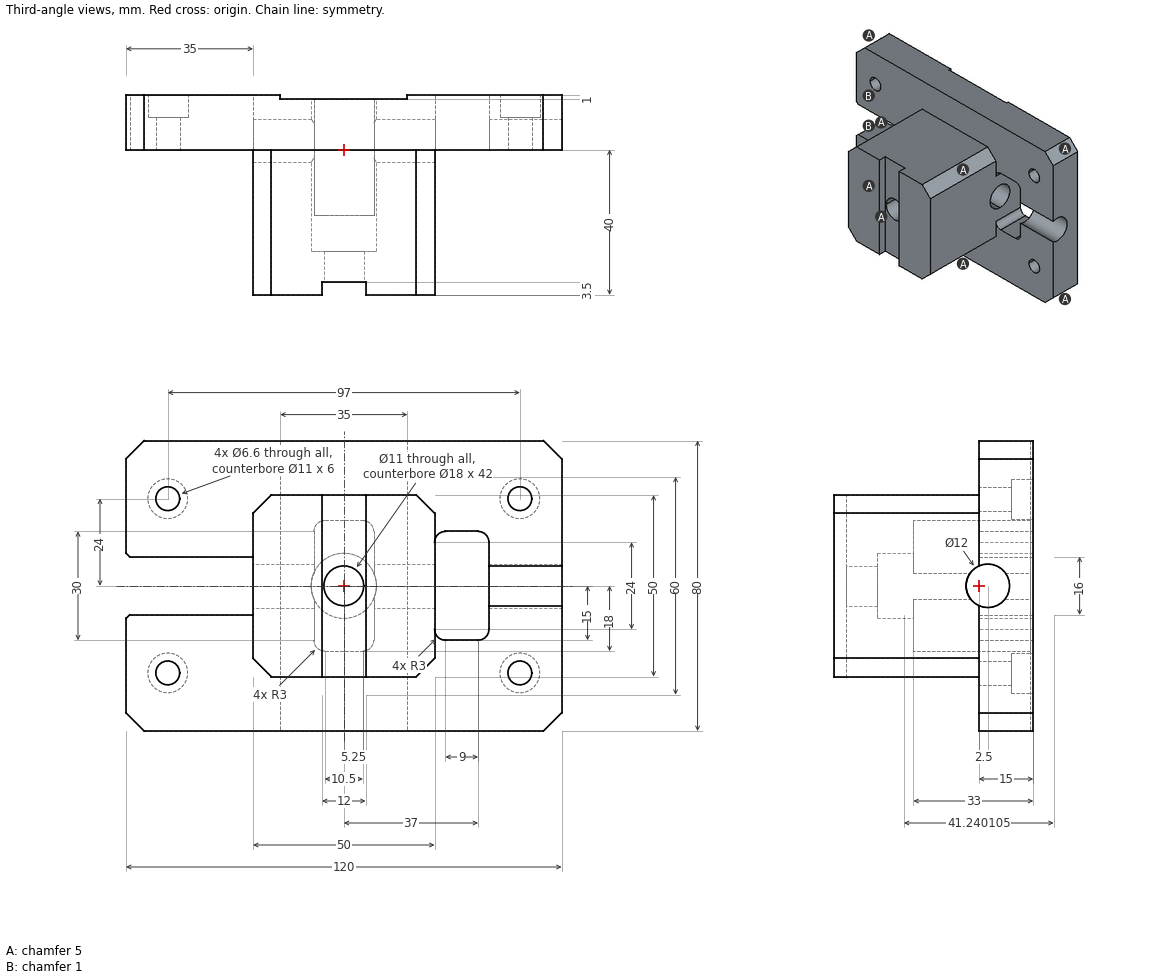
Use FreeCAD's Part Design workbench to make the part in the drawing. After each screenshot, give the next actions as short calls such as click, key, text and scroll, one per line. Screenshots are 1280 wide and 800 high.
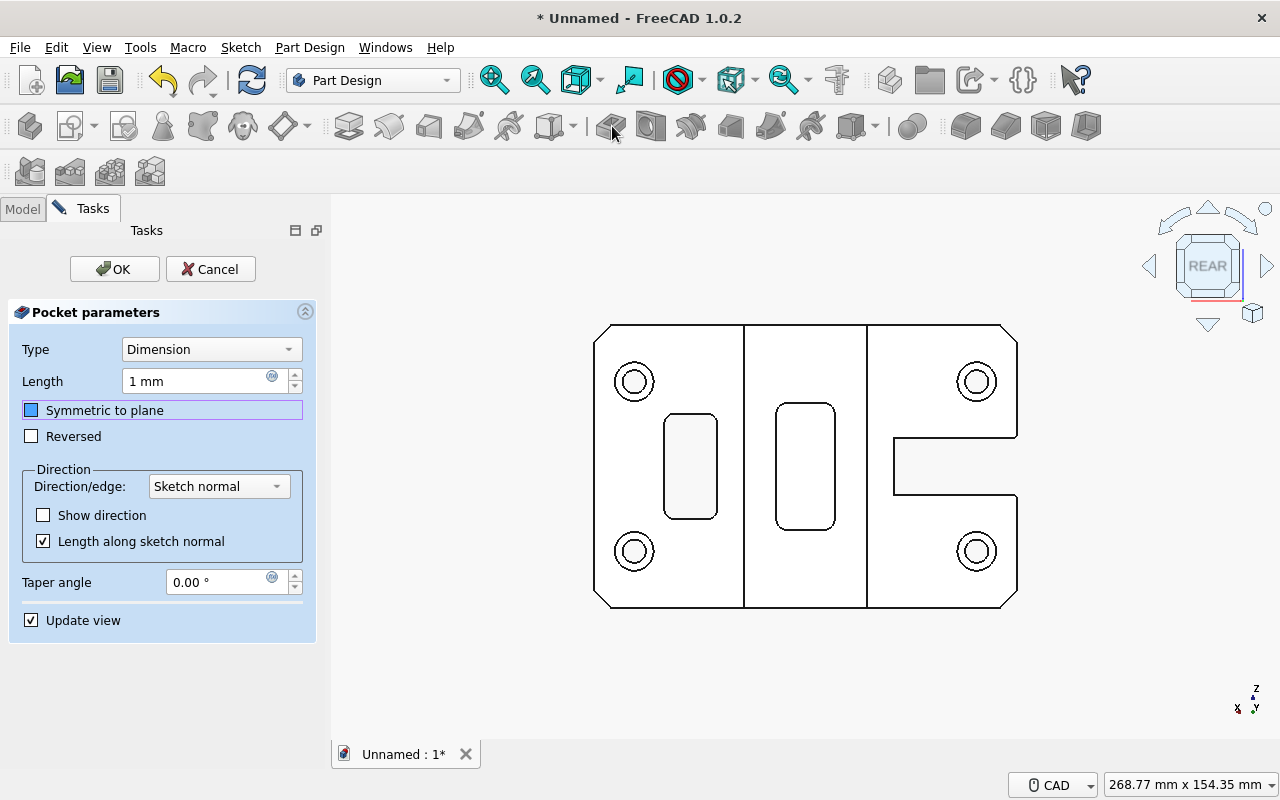
click(115, 269)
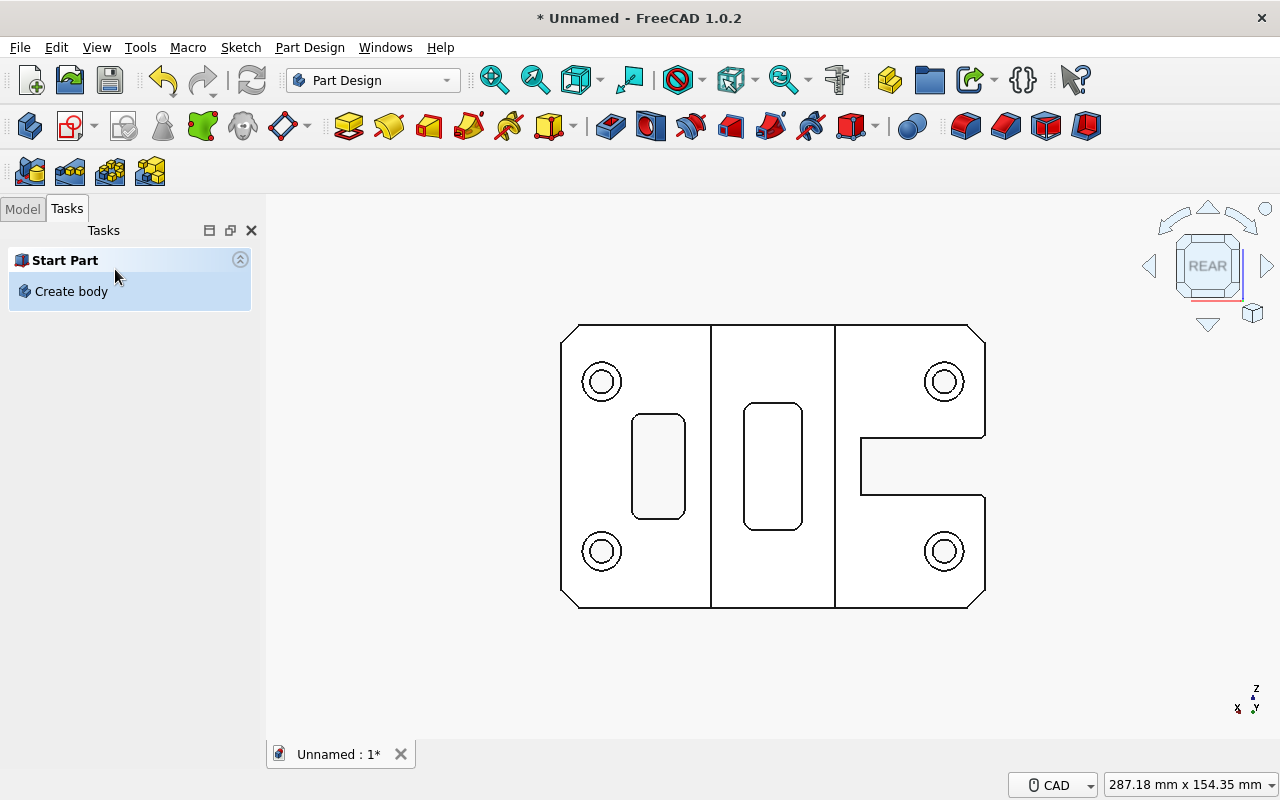
click(738, 546)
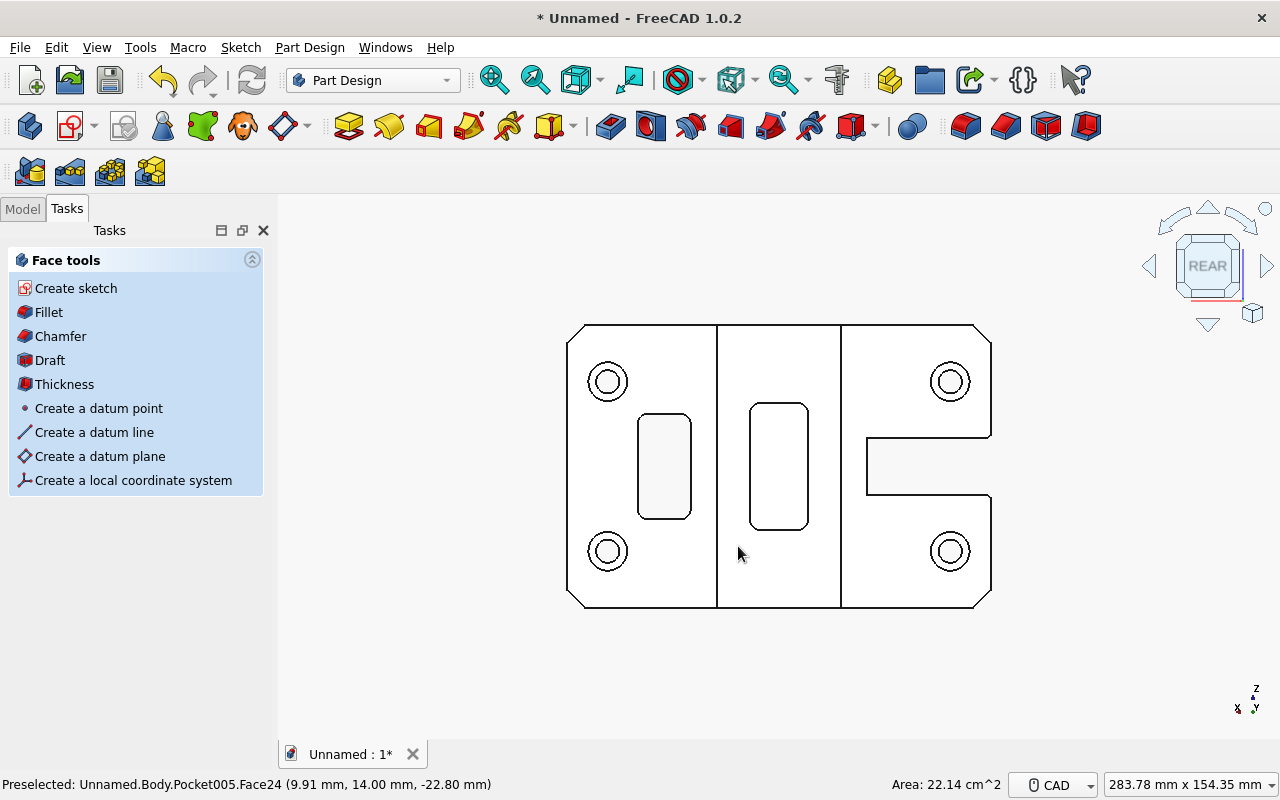
click(70, 126)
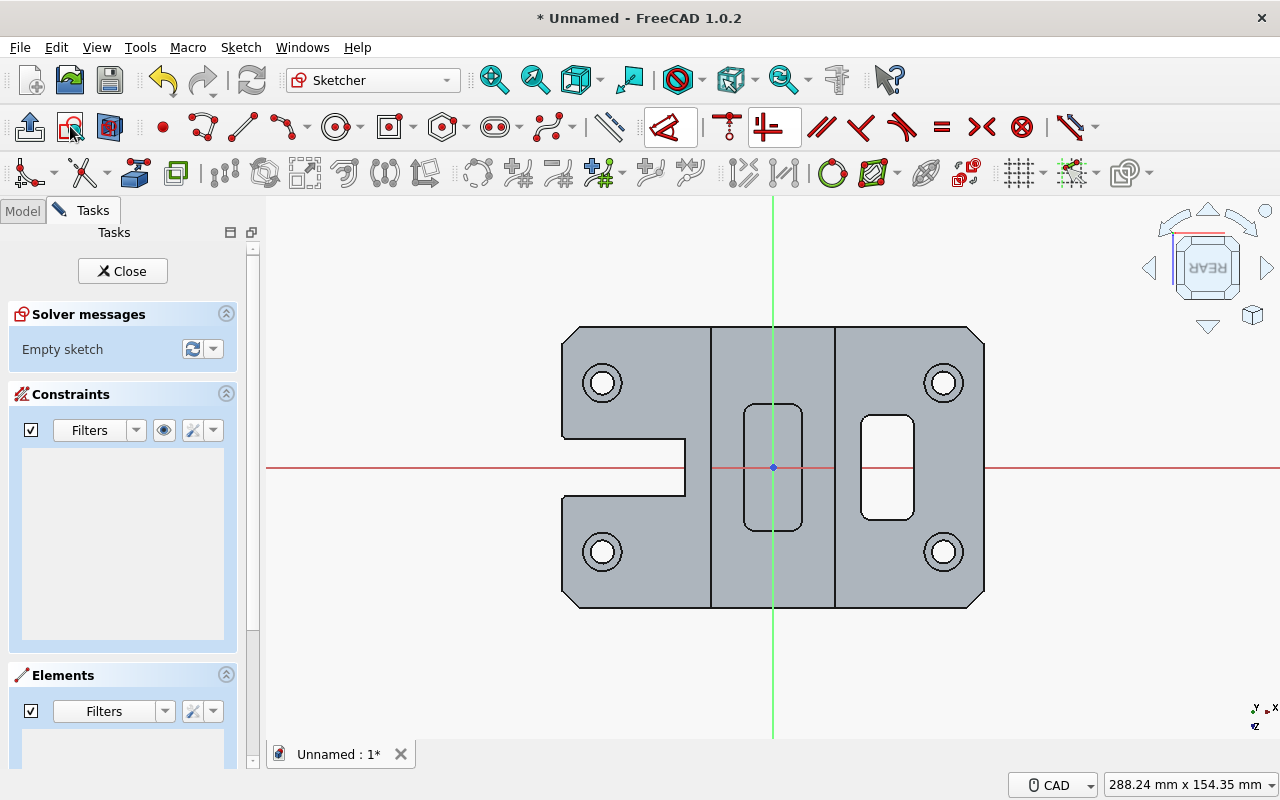
scroll(782, 467, up, 11)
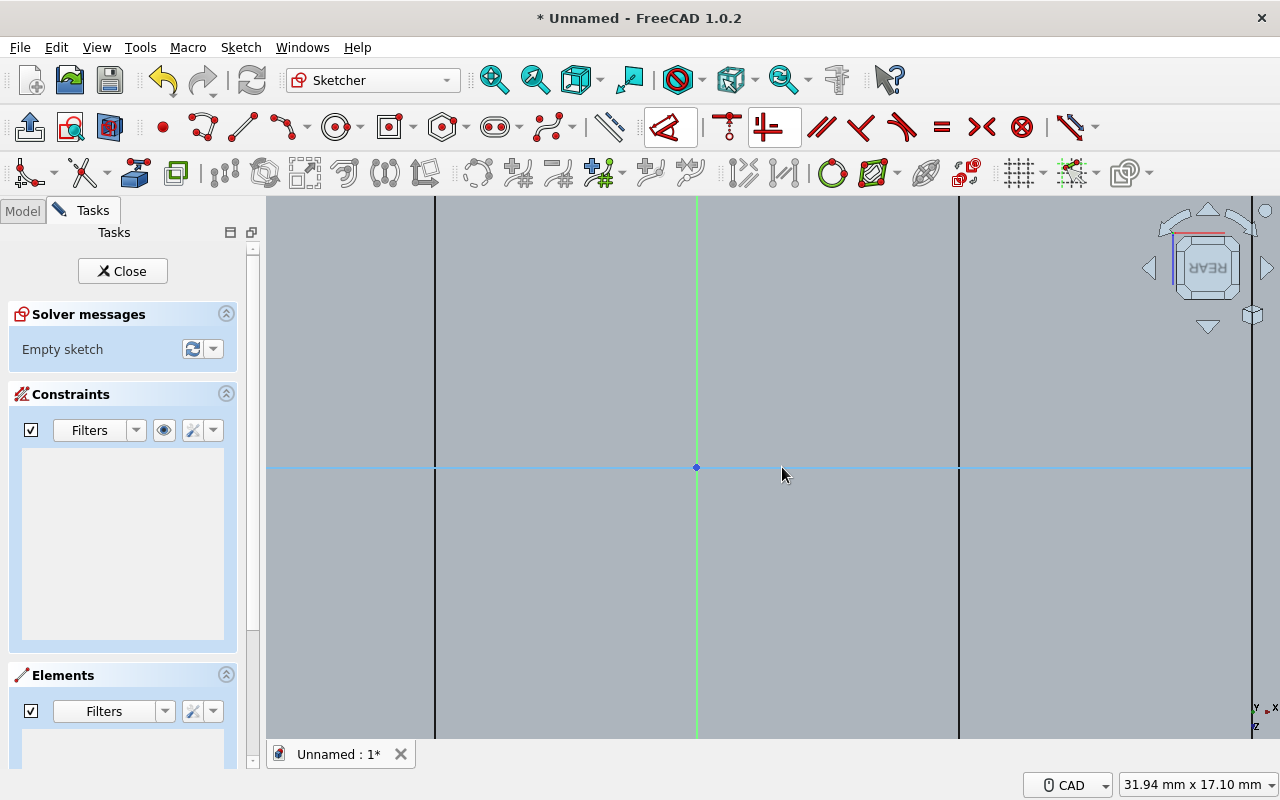
click(336, 128)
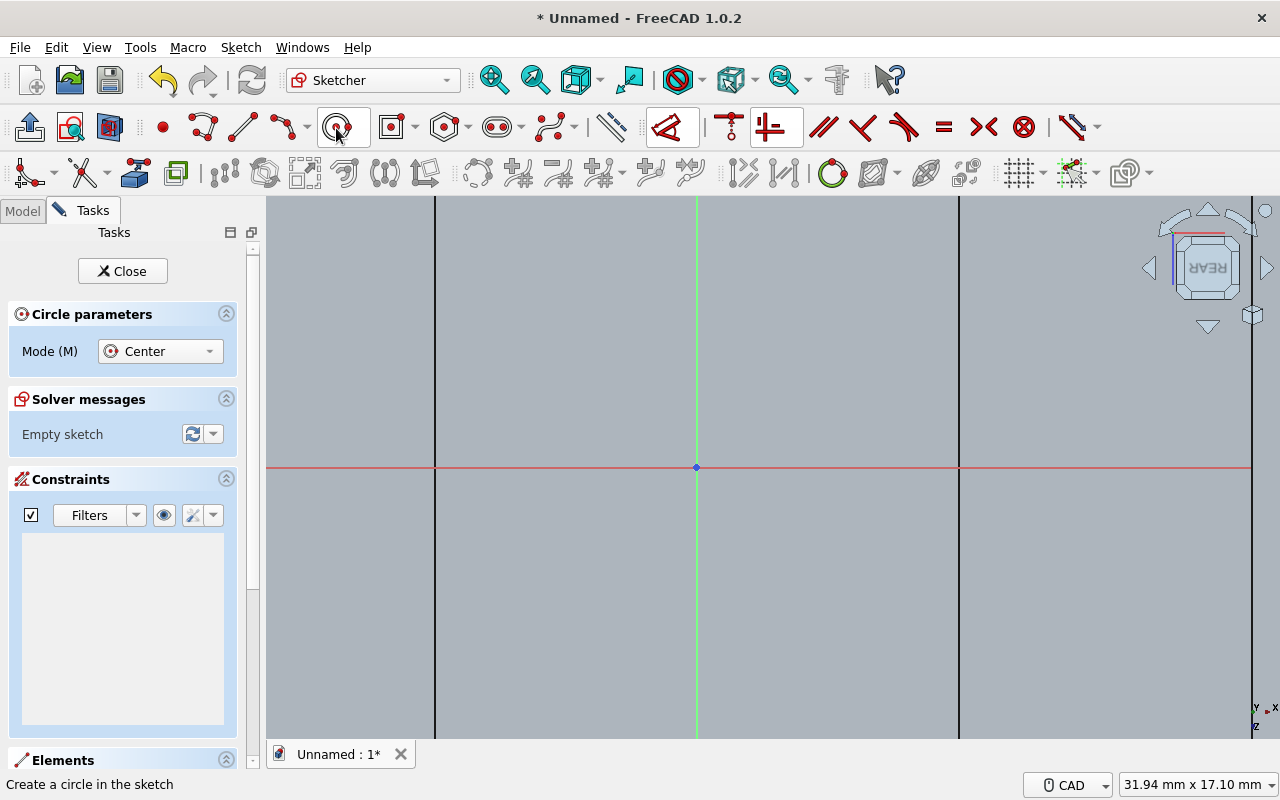
click(697, 467)
click(820, 344)
key(Escape)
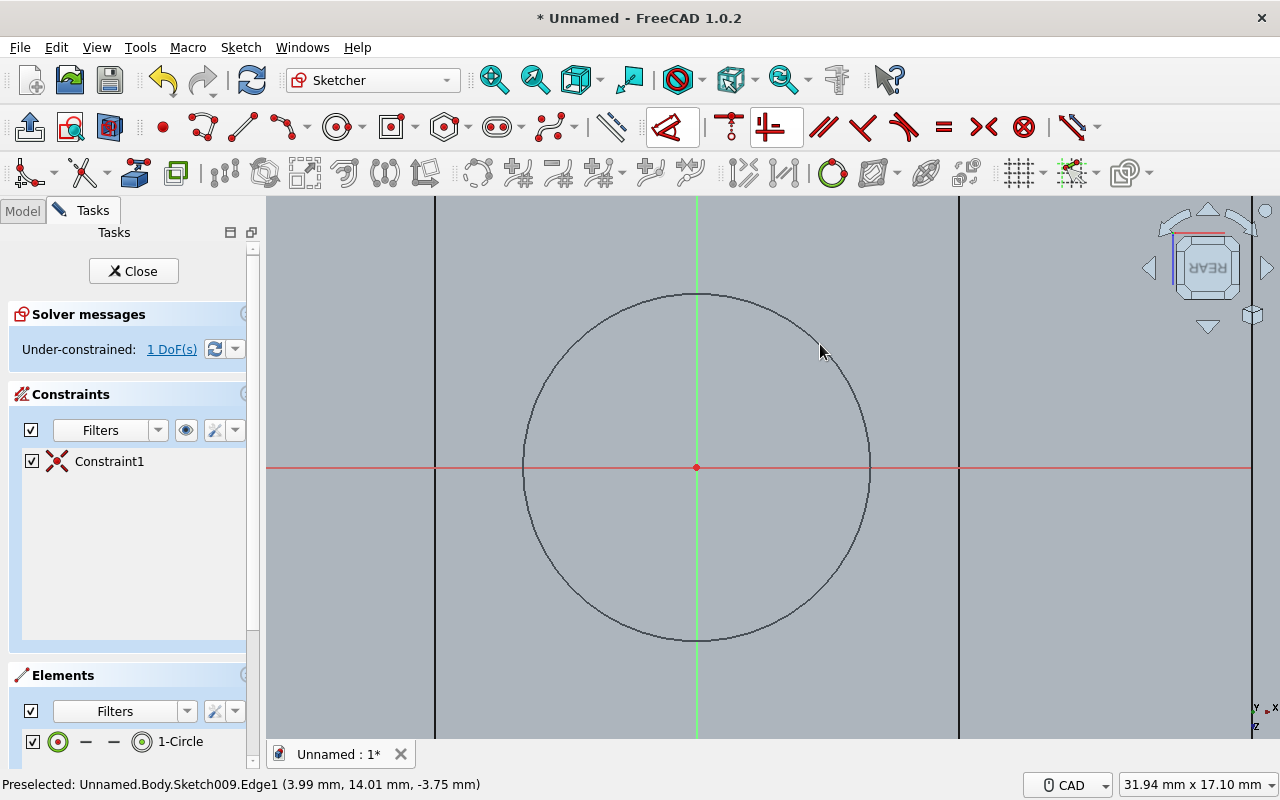
click(819, 344)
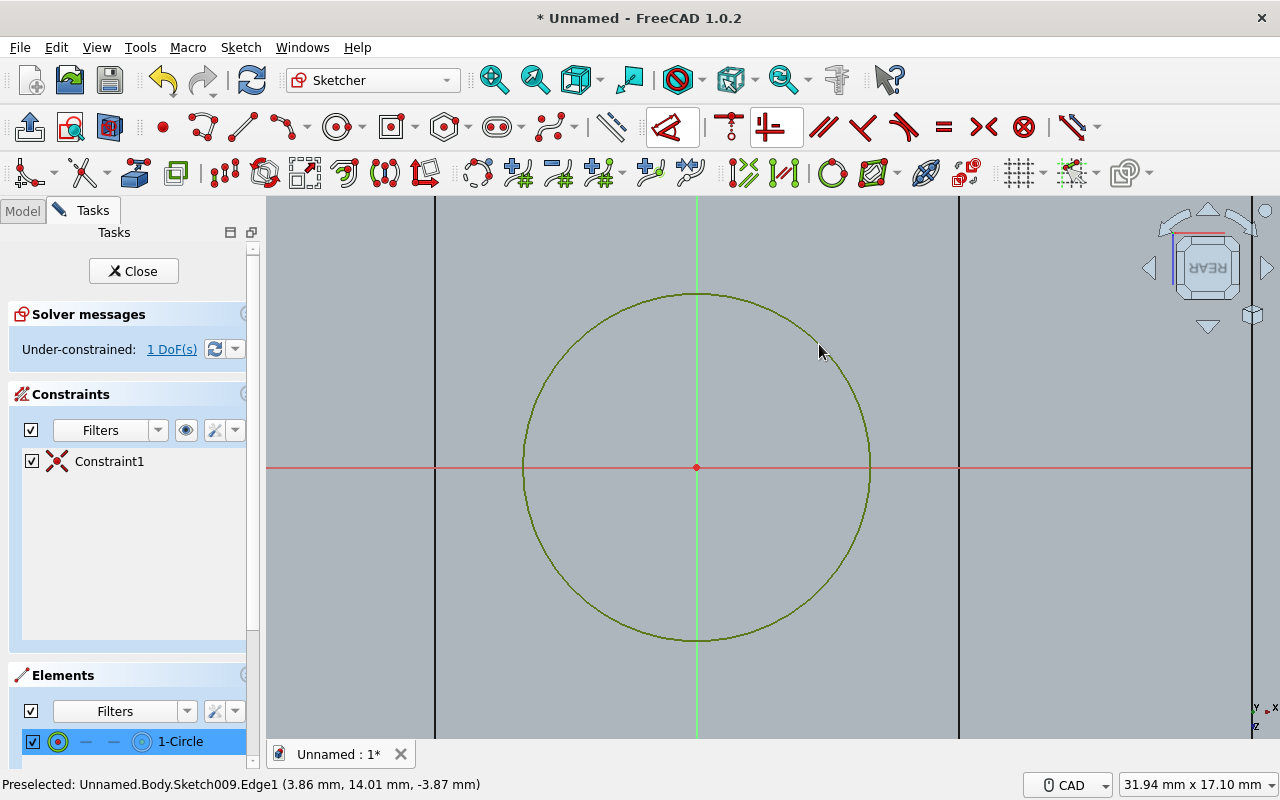
key(k)
key(o)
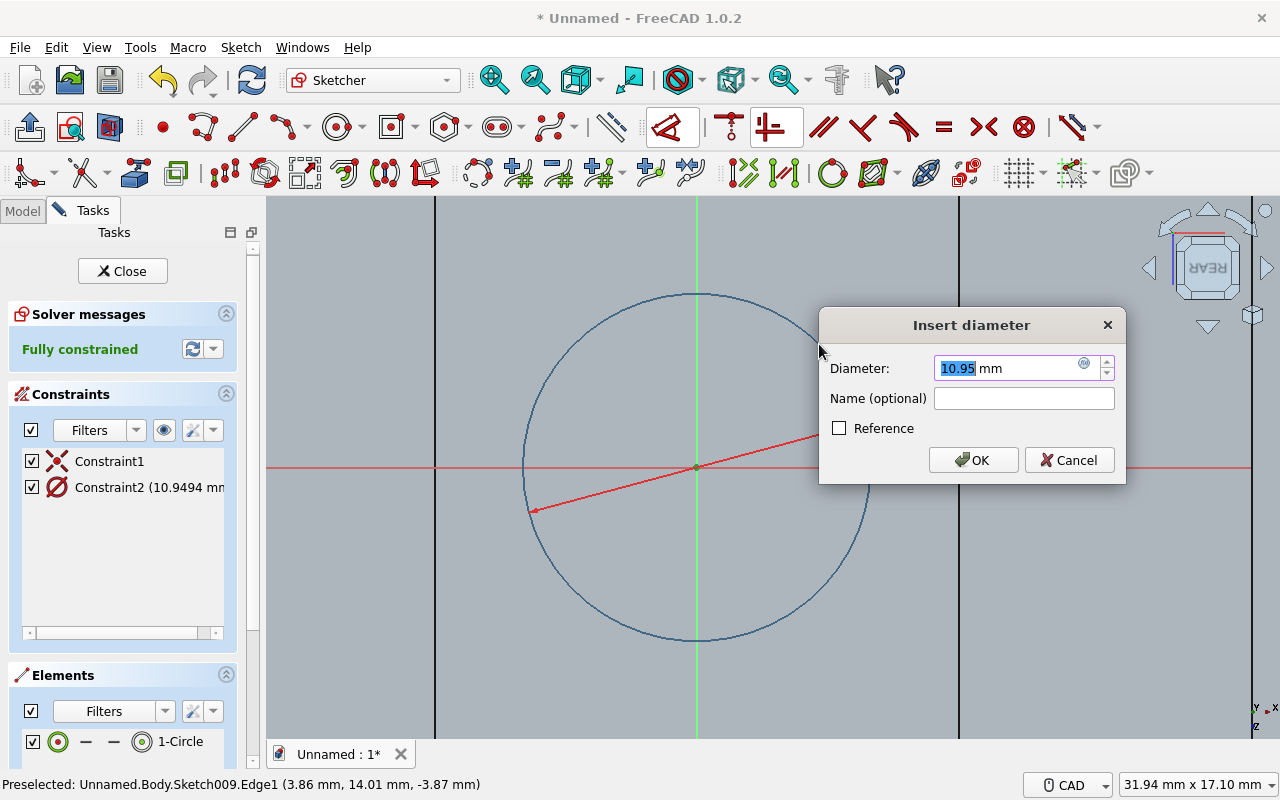
text(11)
key(Return)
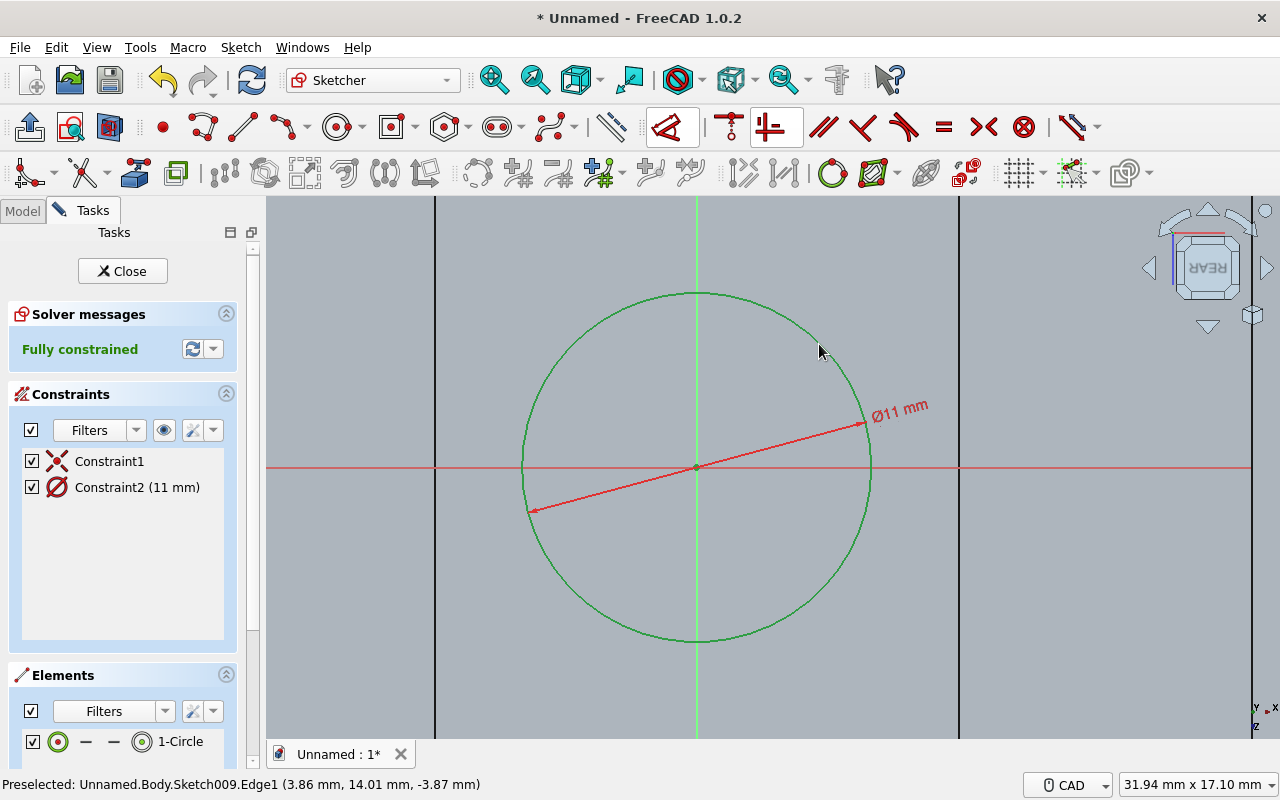
click(123, 271)